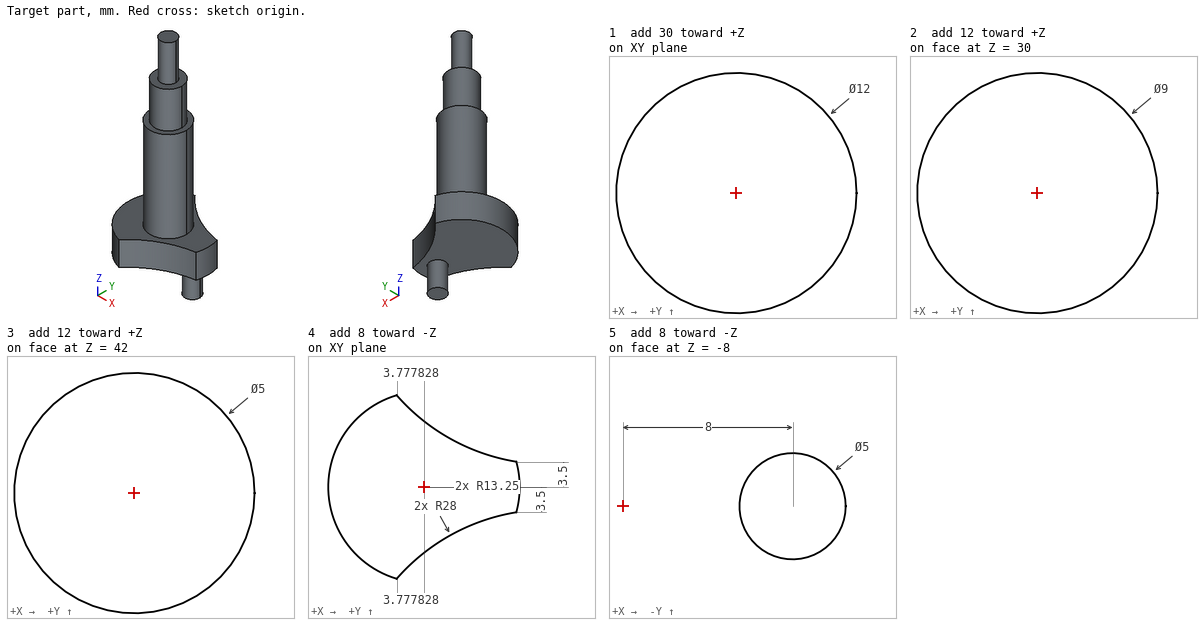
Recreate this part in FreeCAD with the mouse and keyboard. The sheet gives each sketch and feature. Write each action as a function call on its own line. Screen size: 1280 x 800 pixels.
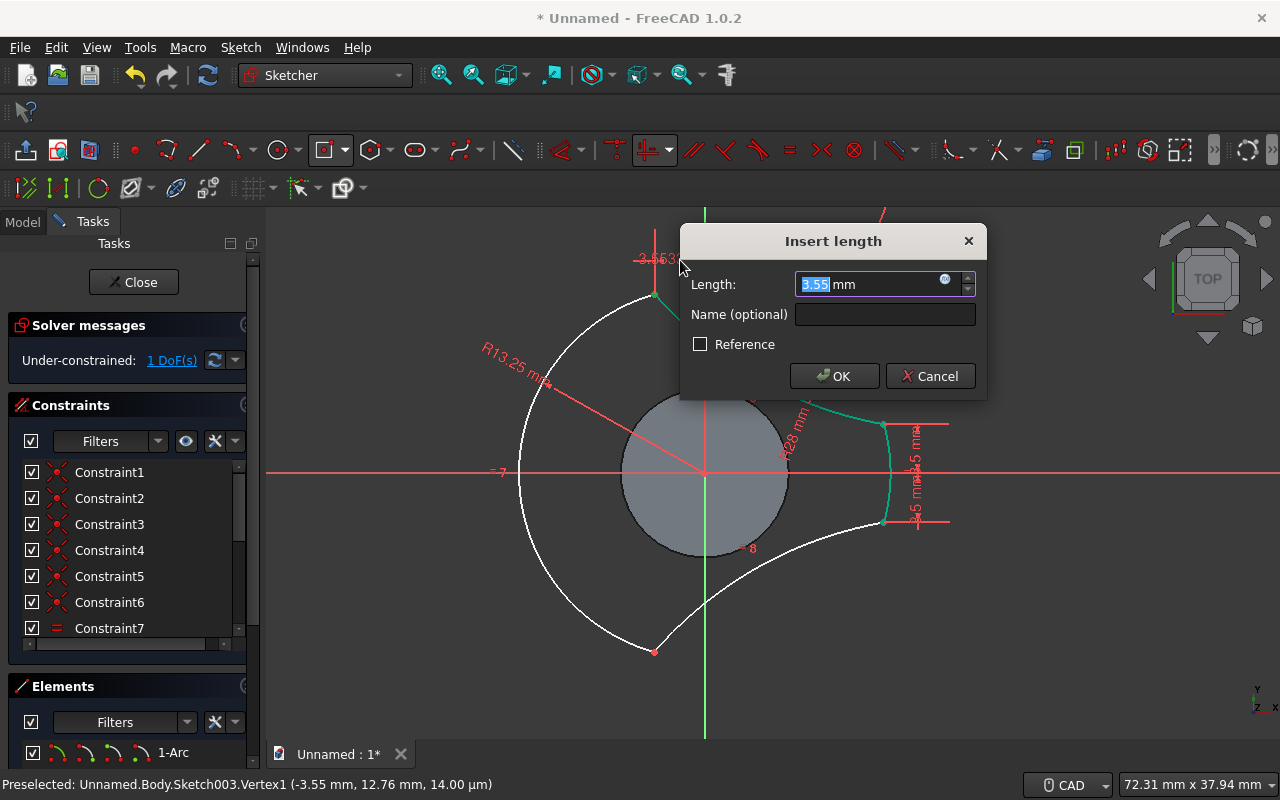
text(3.777828)
key(Return)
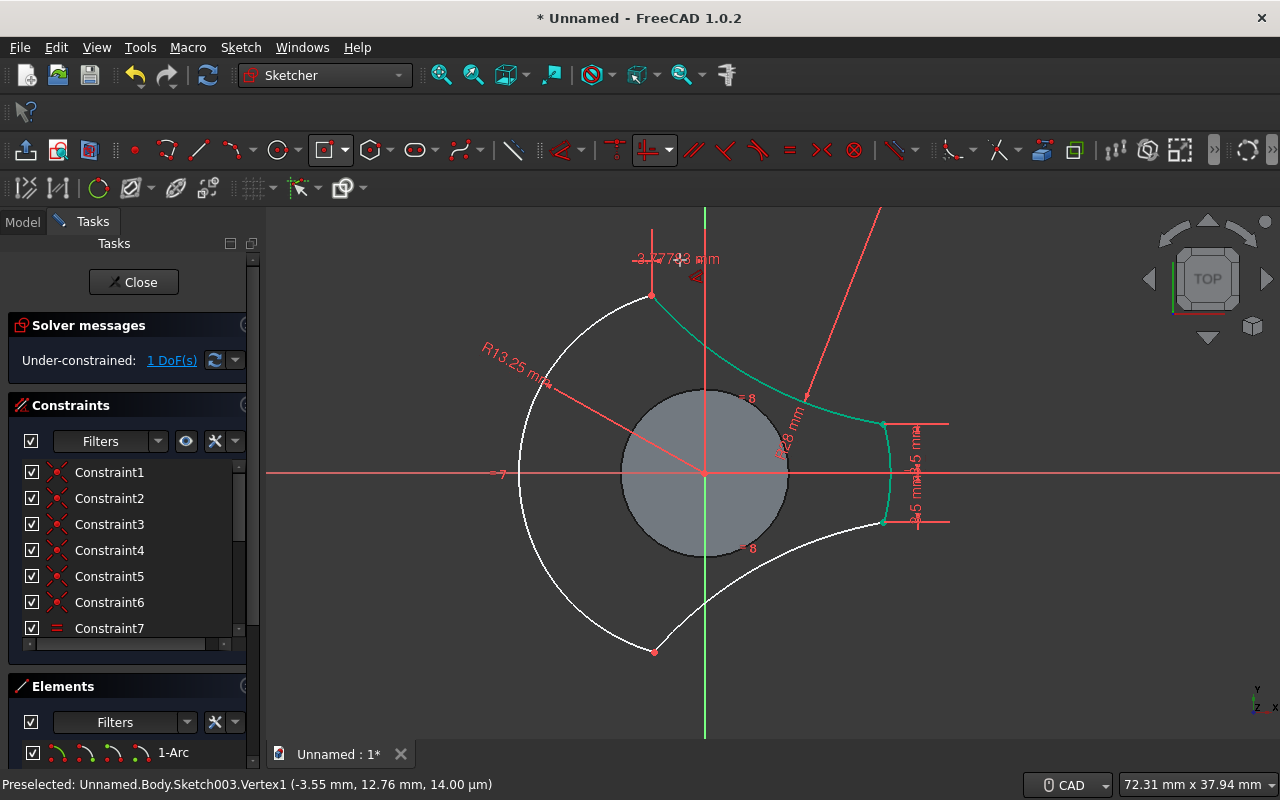
click(654, 652)
click(679, 686)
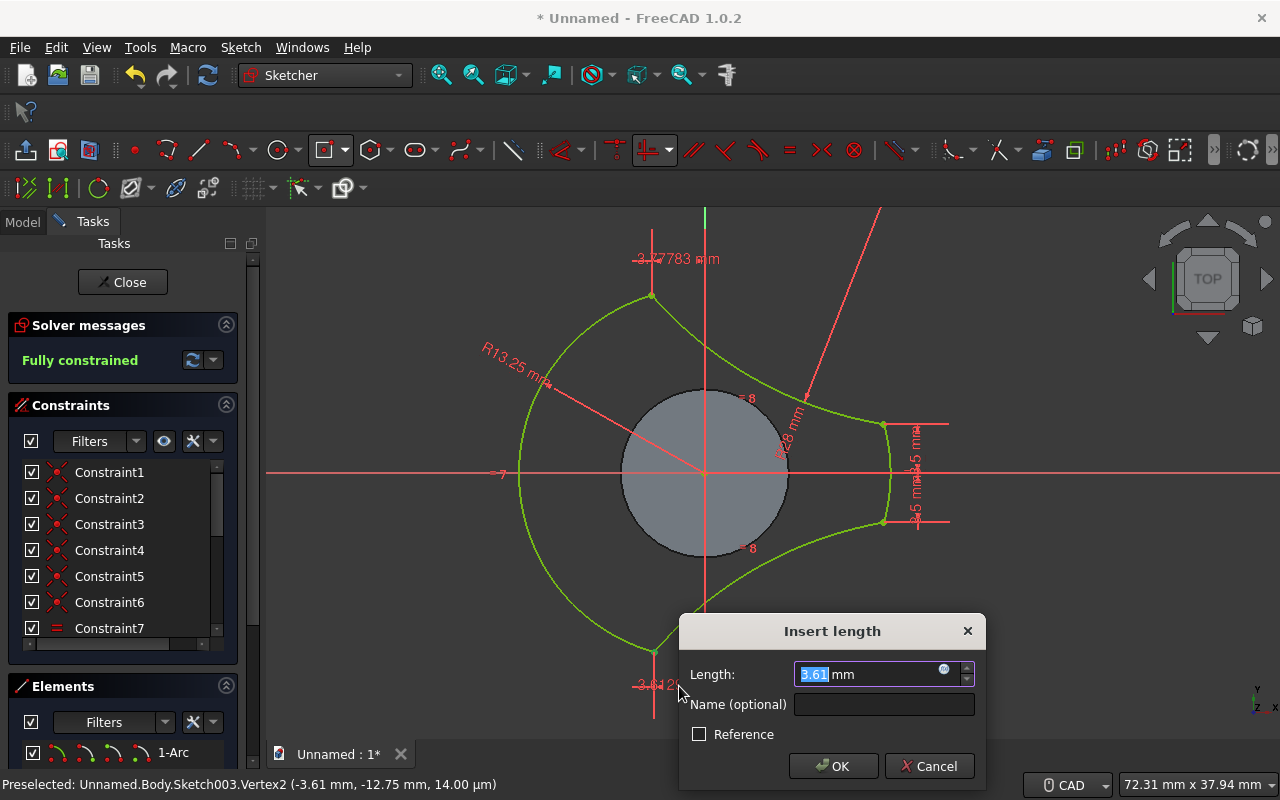
text(3.777828)
key(Return)
key(Escape)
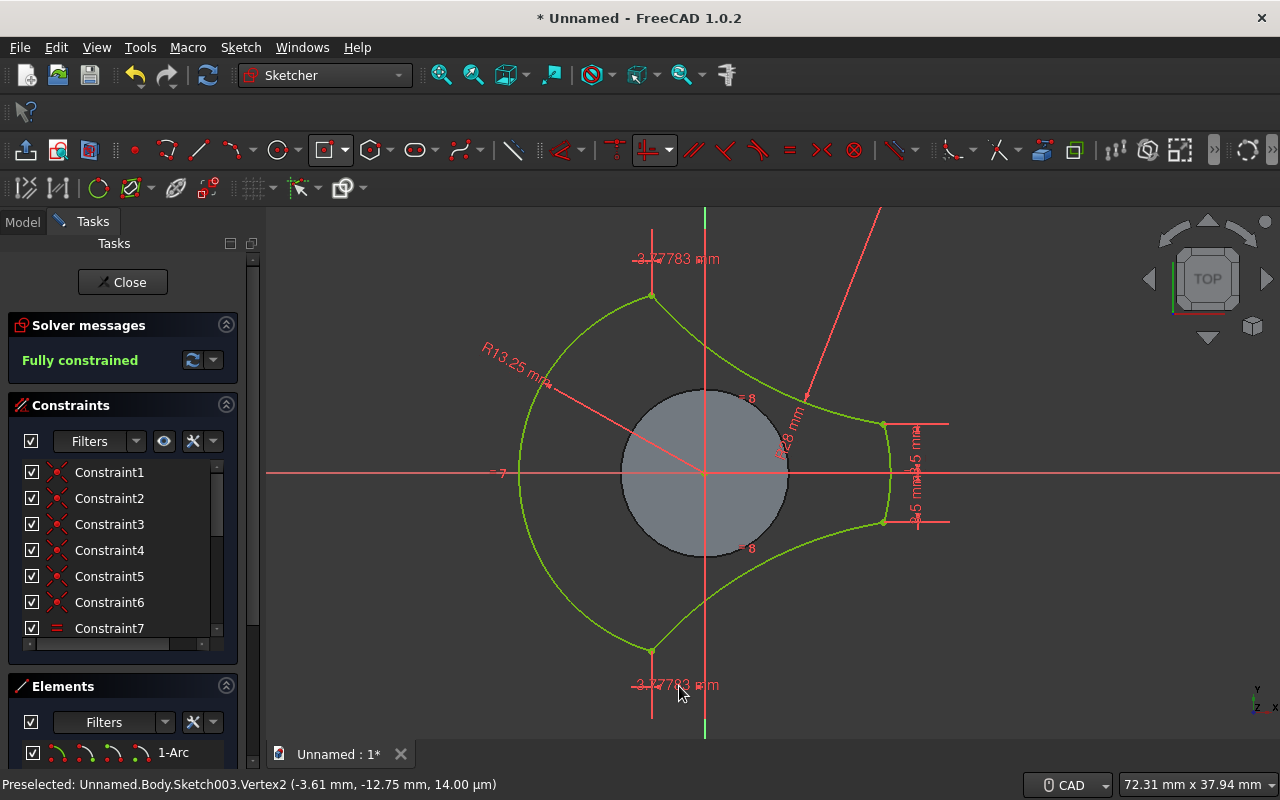
click(123, 282)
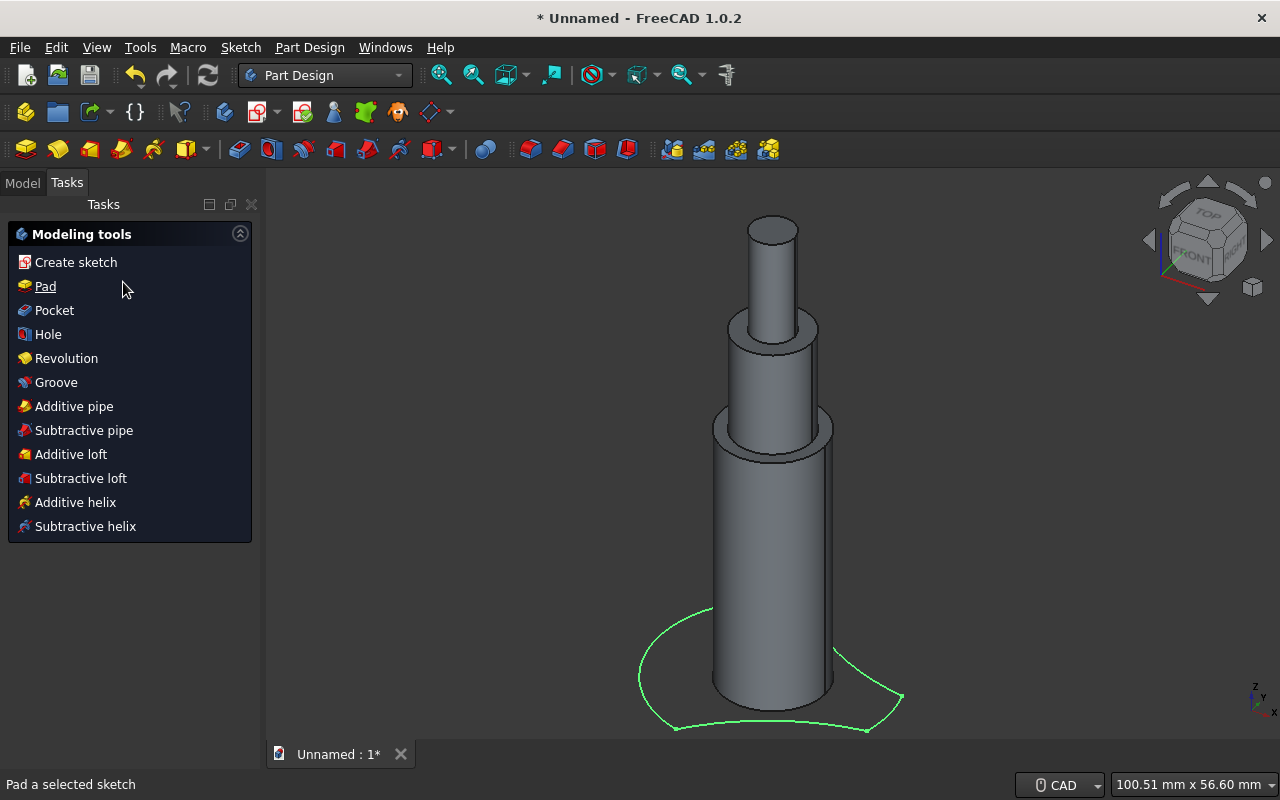
click(26, 150)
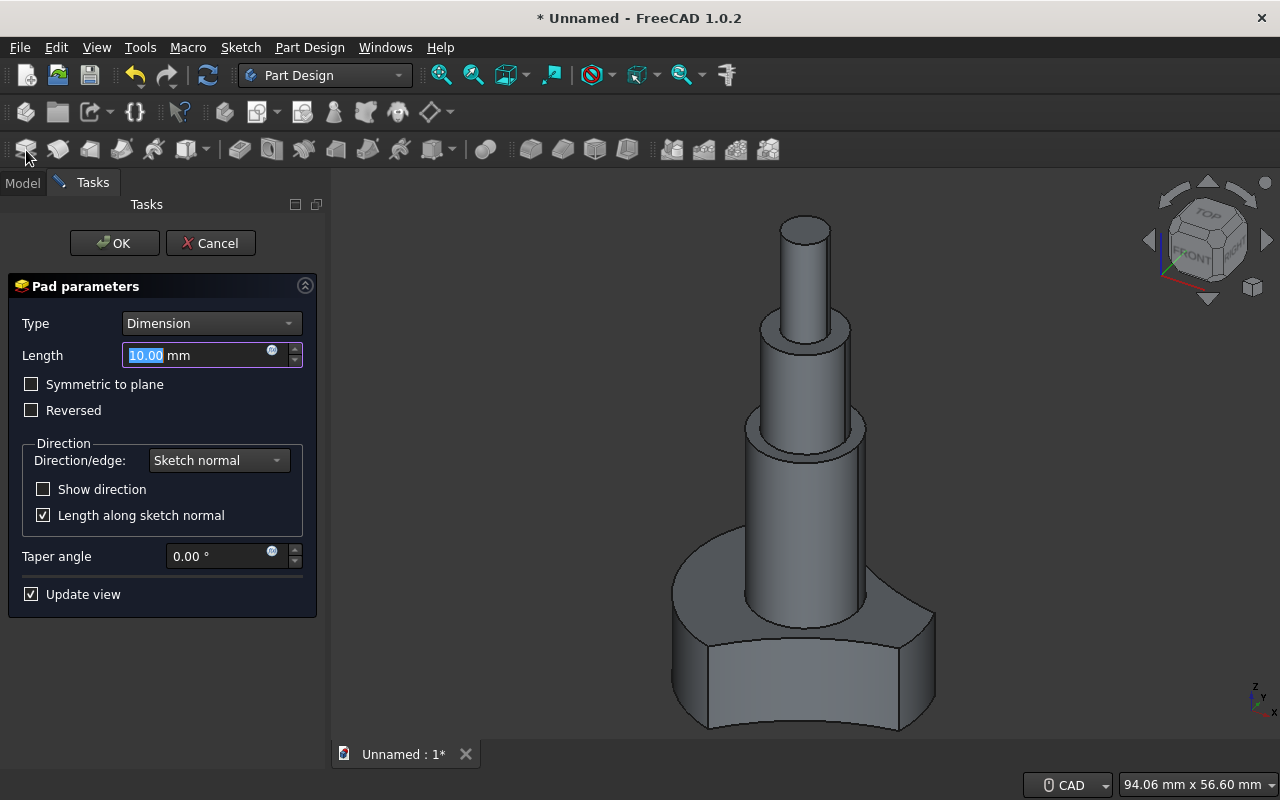
text(8)
key(Tab)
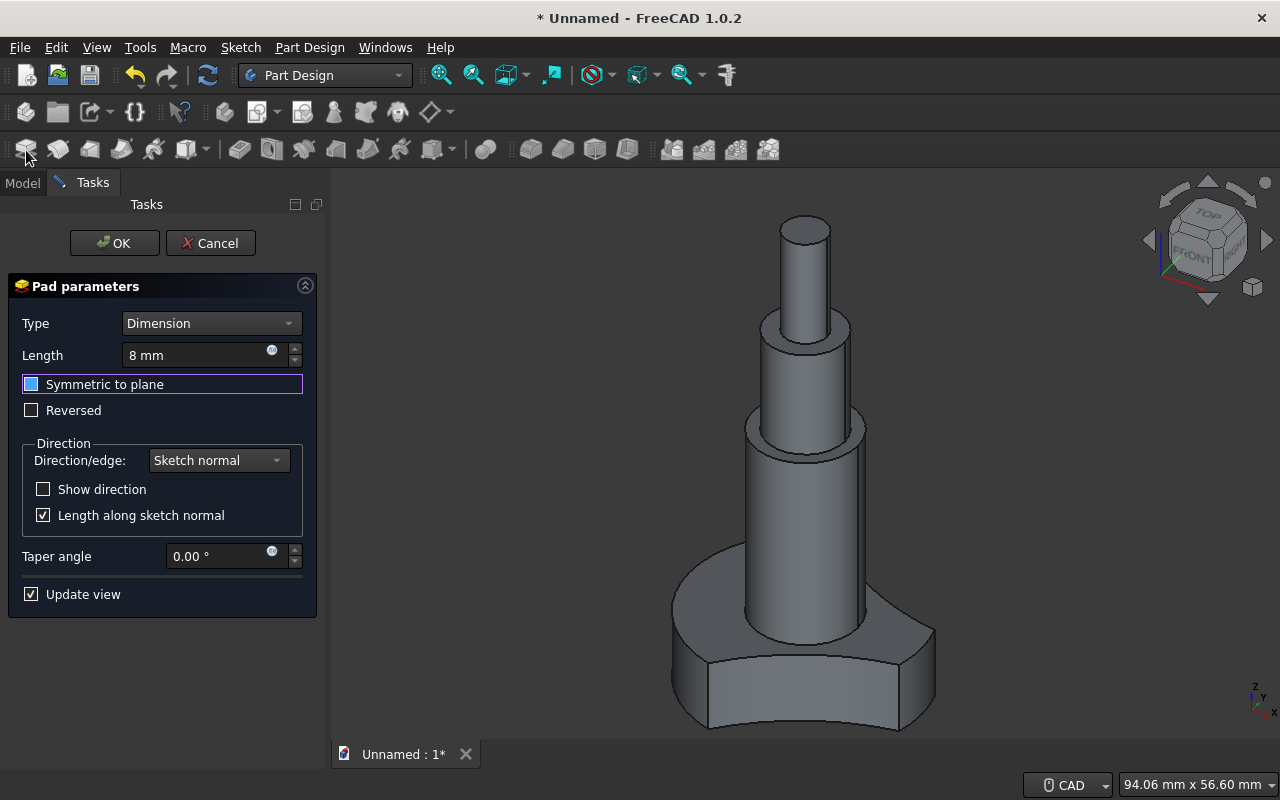
click(30, 410)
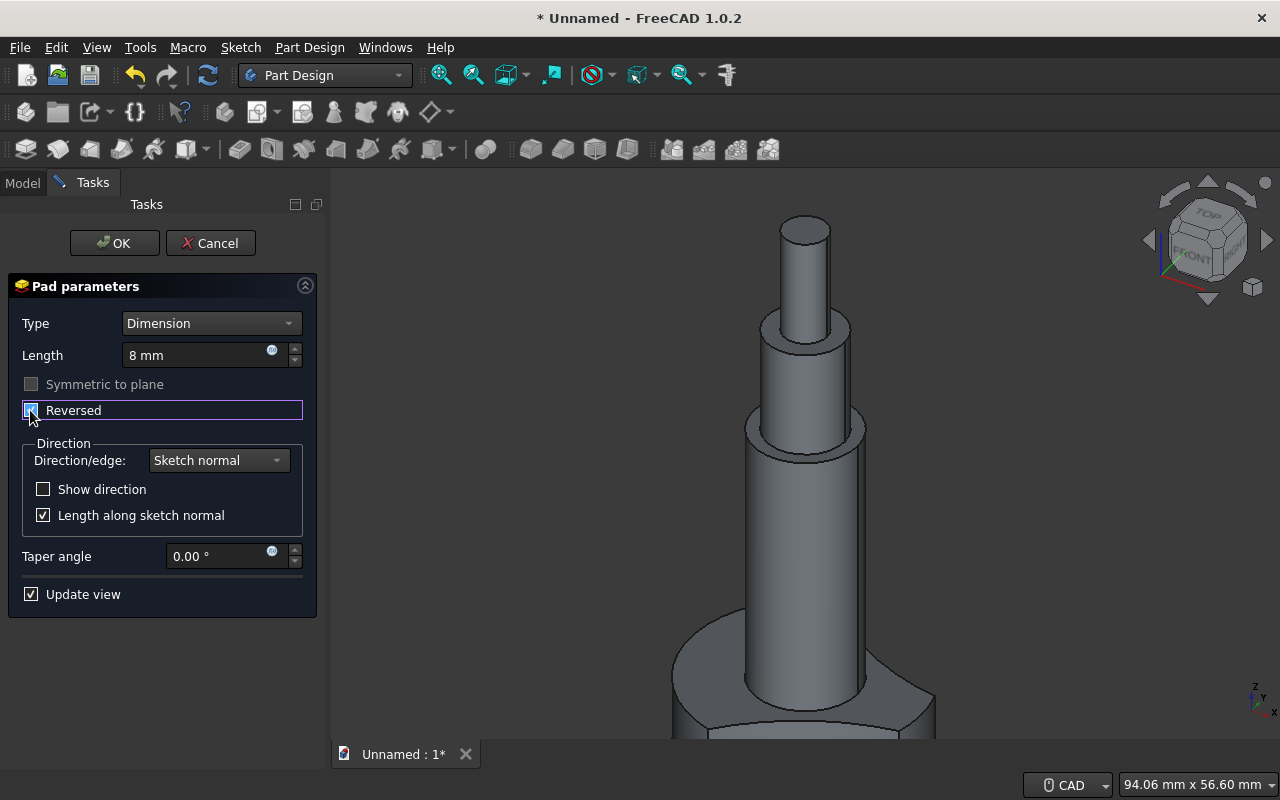
click(115, 243)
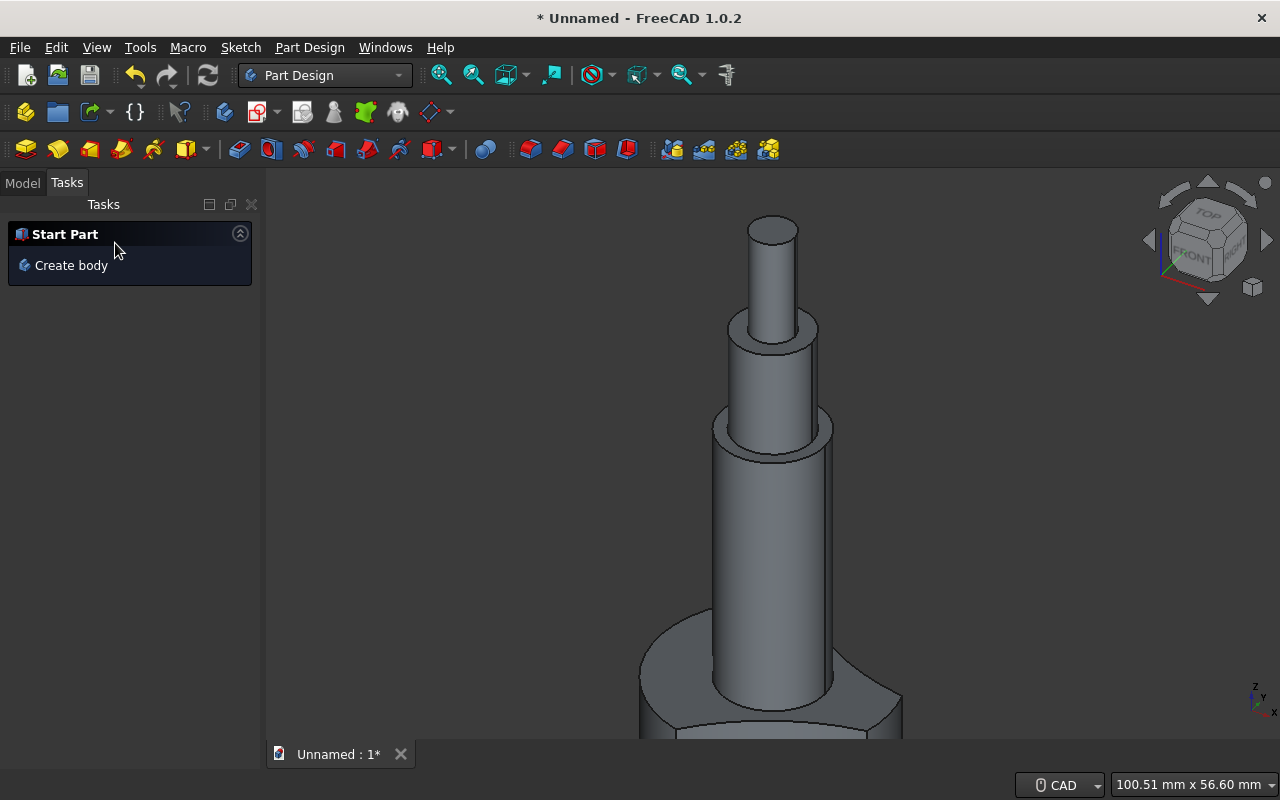
click(442, 76)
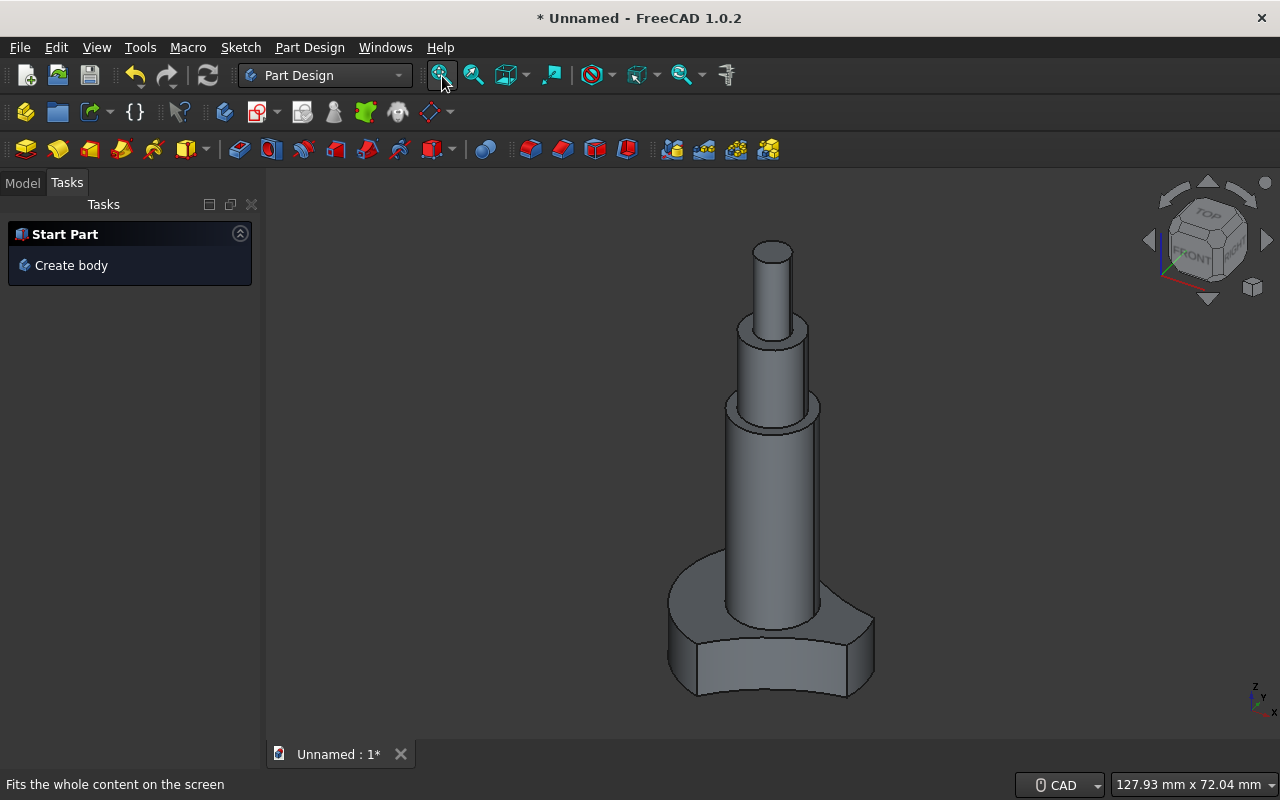
key(5)